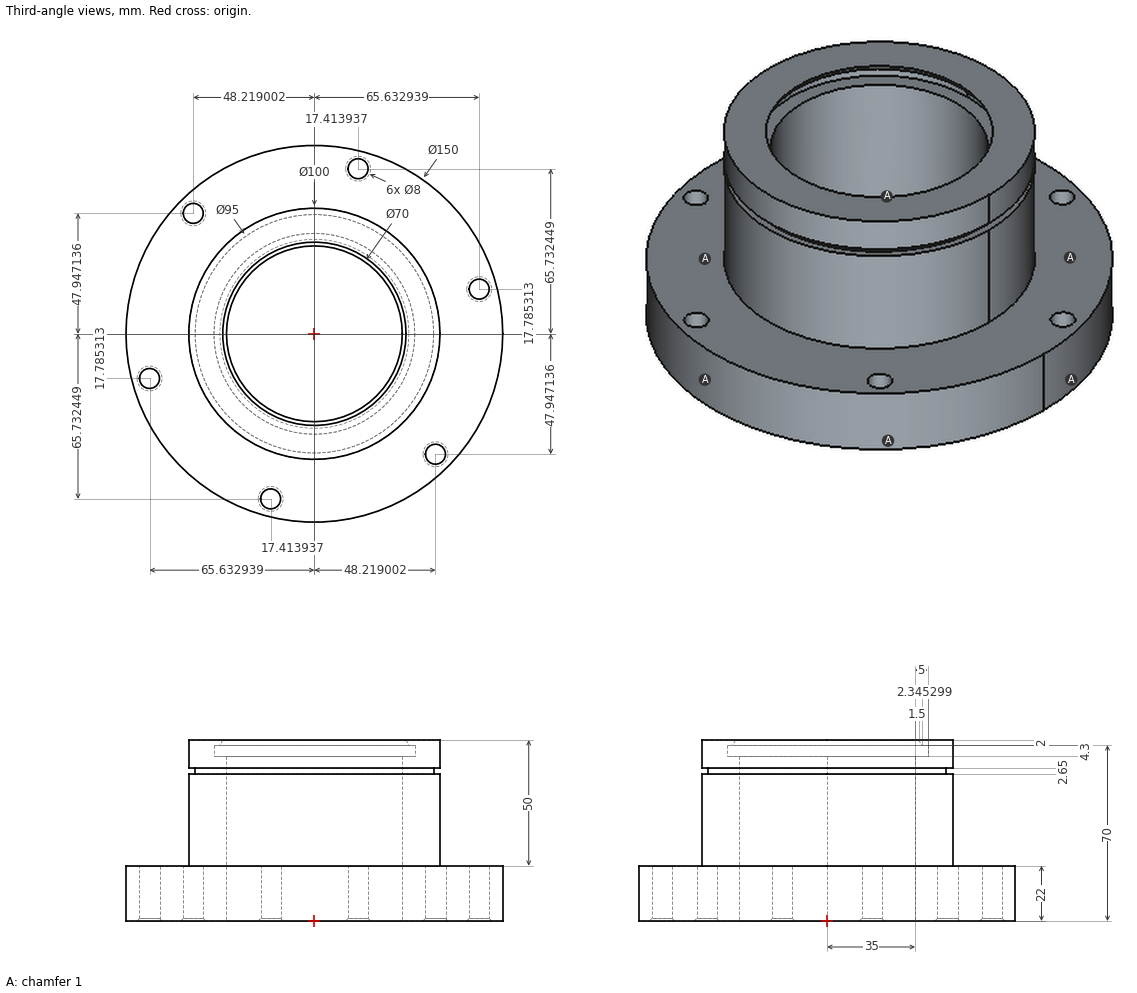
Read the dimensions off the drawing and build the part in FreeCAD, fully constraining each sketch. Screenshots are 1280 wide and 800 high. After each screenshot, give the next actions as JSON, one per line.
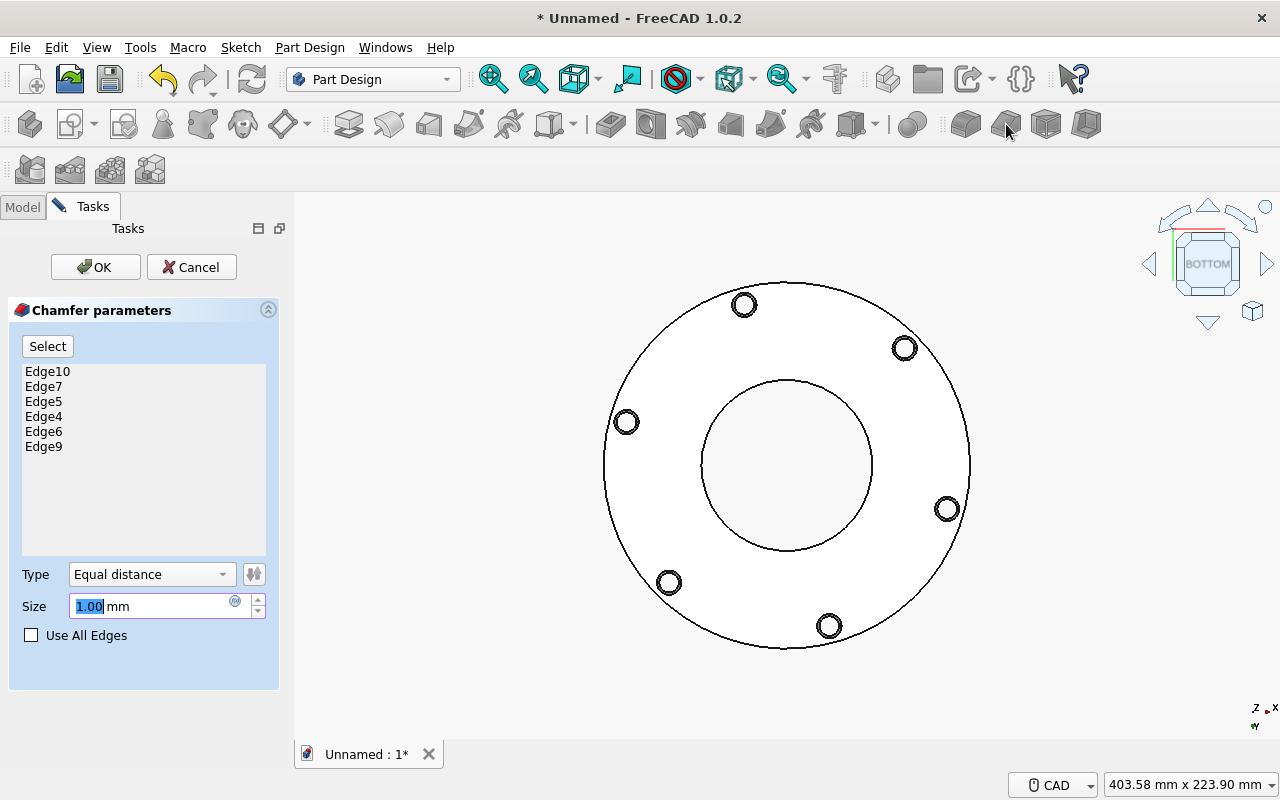
{"action": "type", "text": "1"}
{"action": "key", "text": "Tab"}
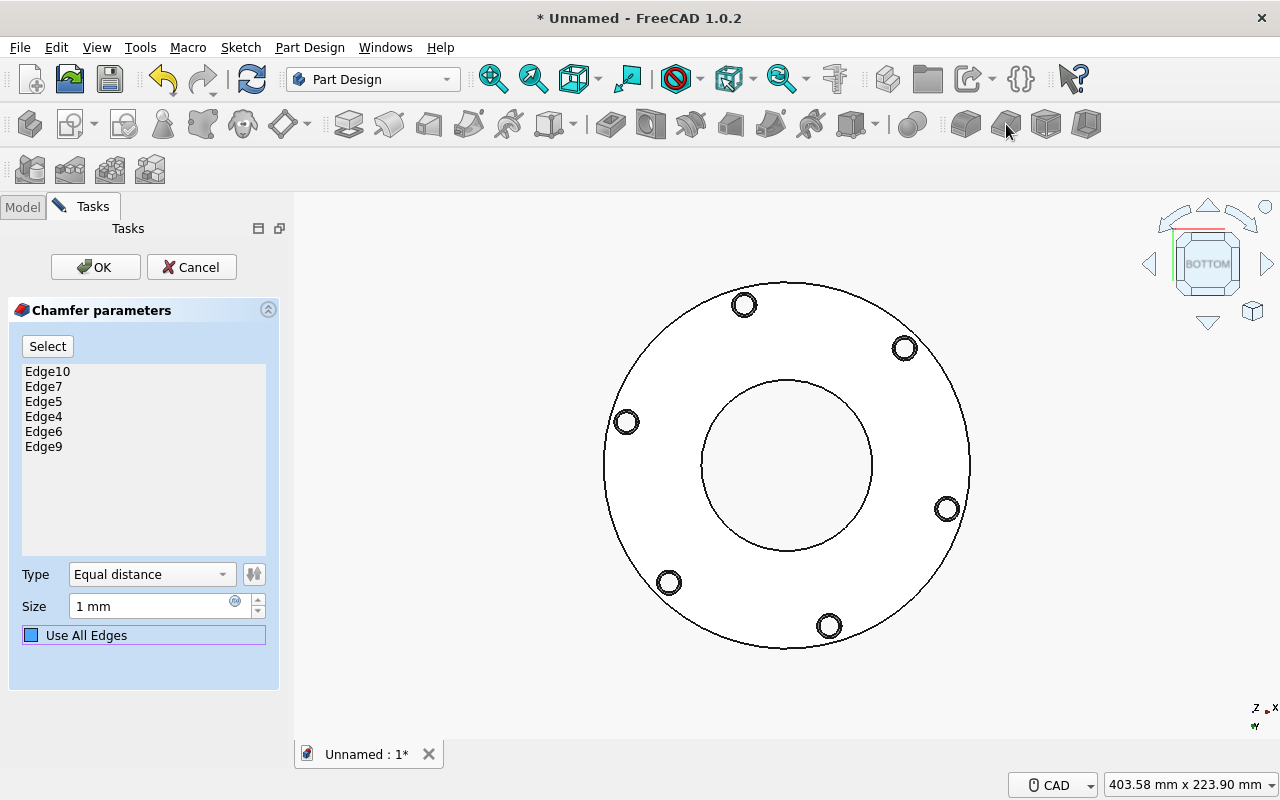
{"action": "left_click", "coordinate": [96, 267]}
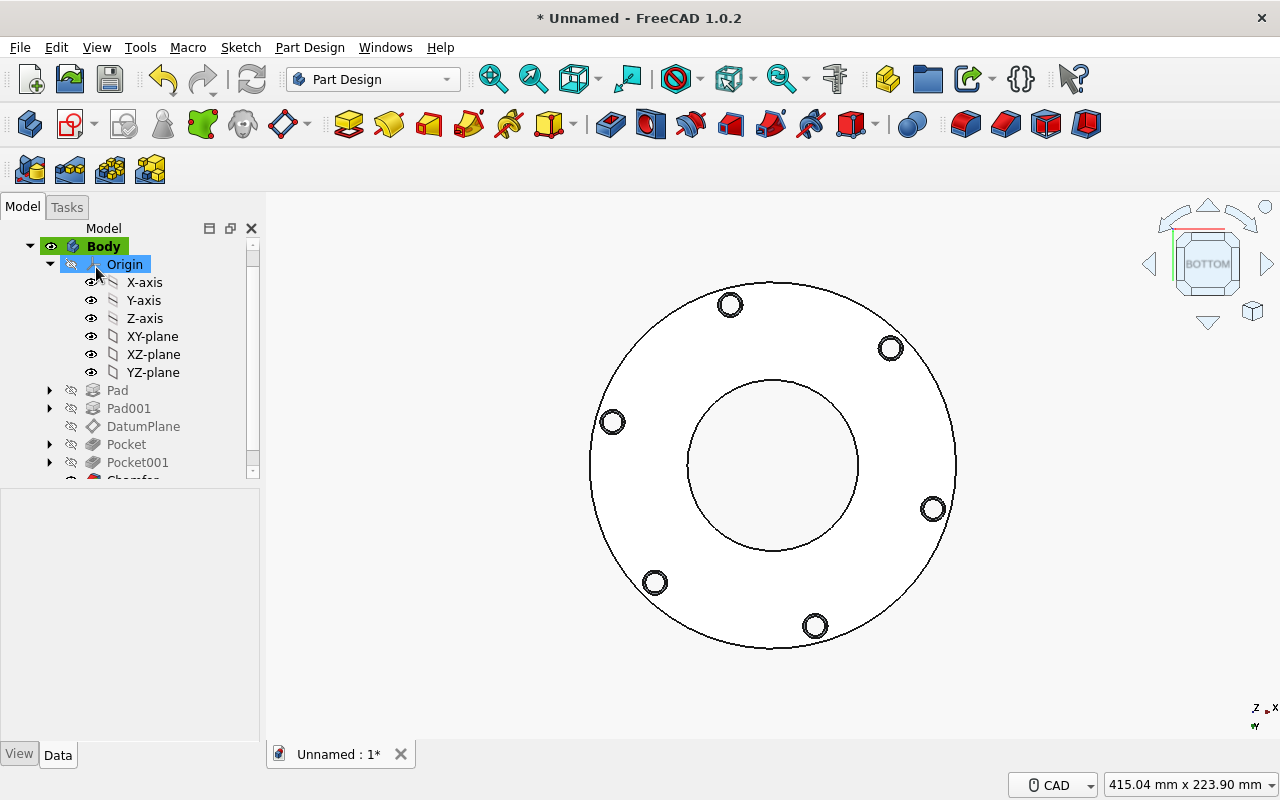
{"action": "left_click", "coordinate": [70, 124]}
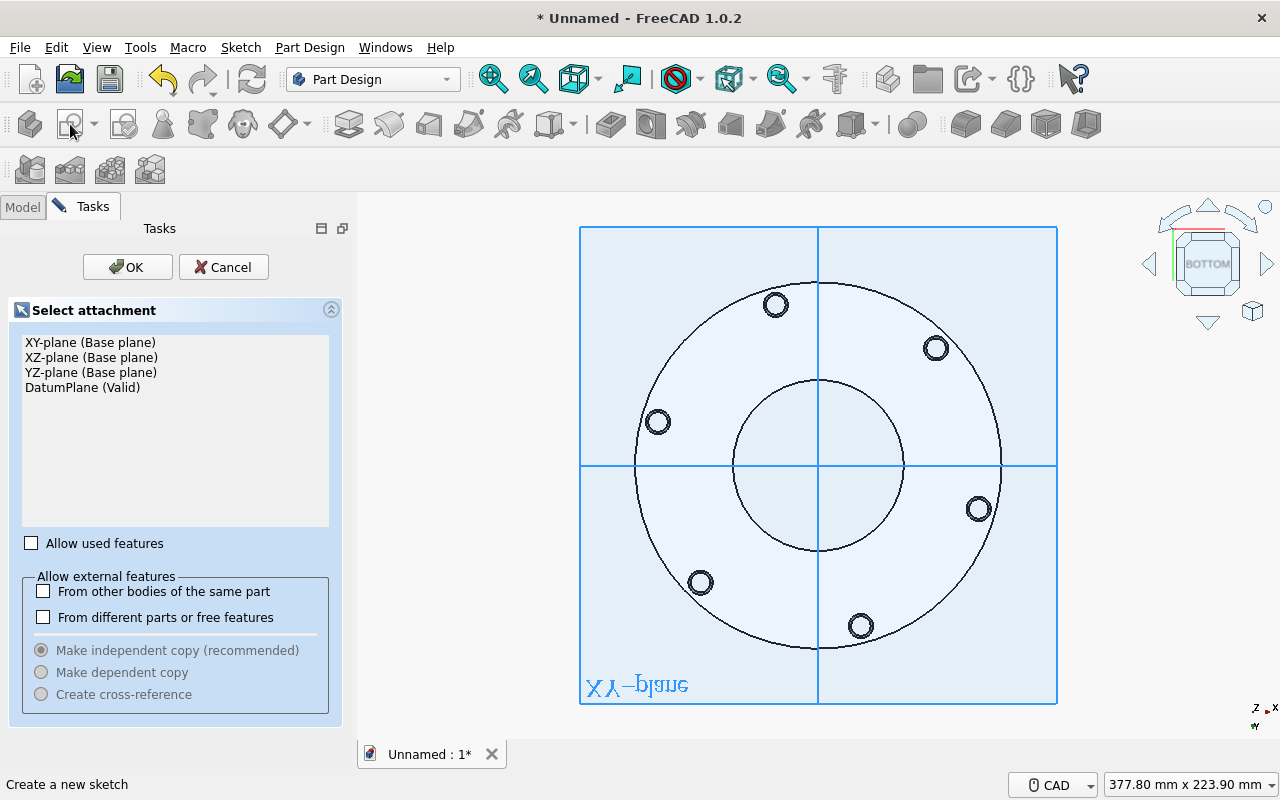
{"action": "left_click", "coordinate": [82, 372]}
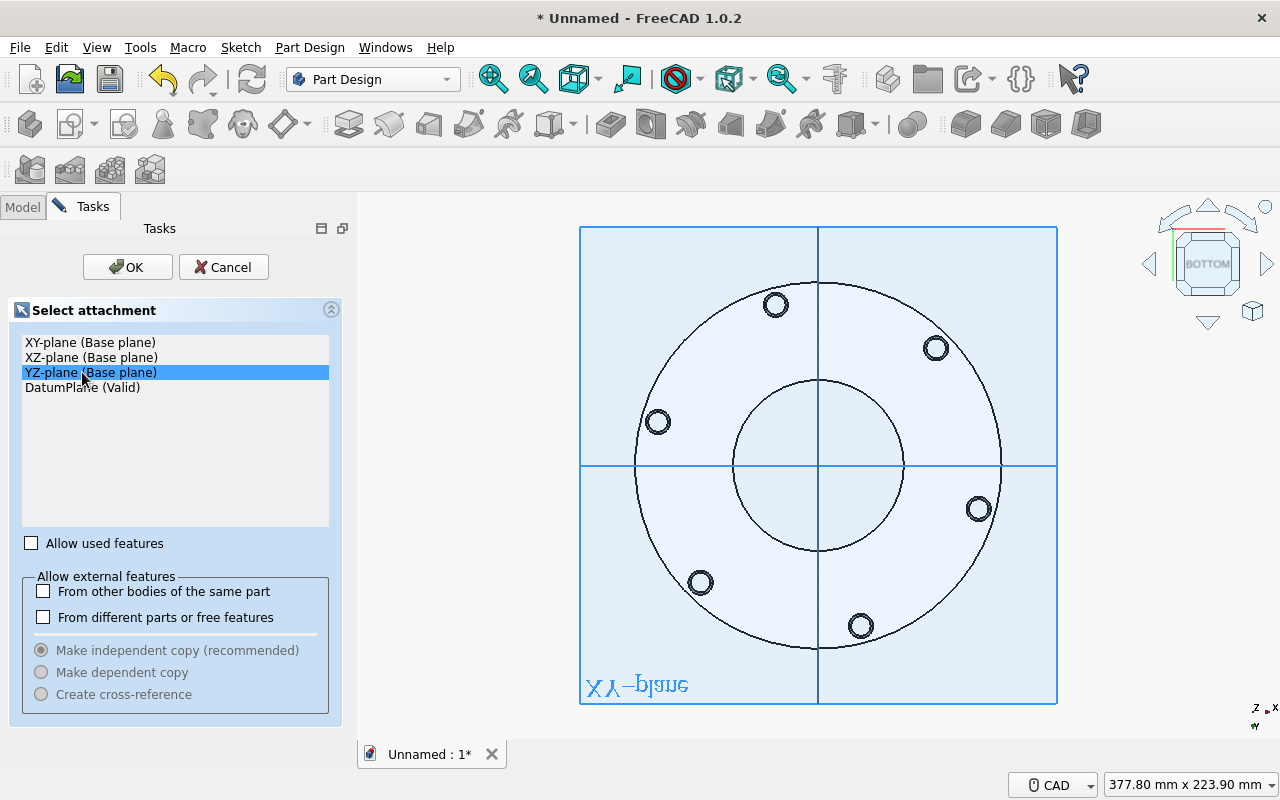
{"action": "left_click", "coordinate": [128, 267]}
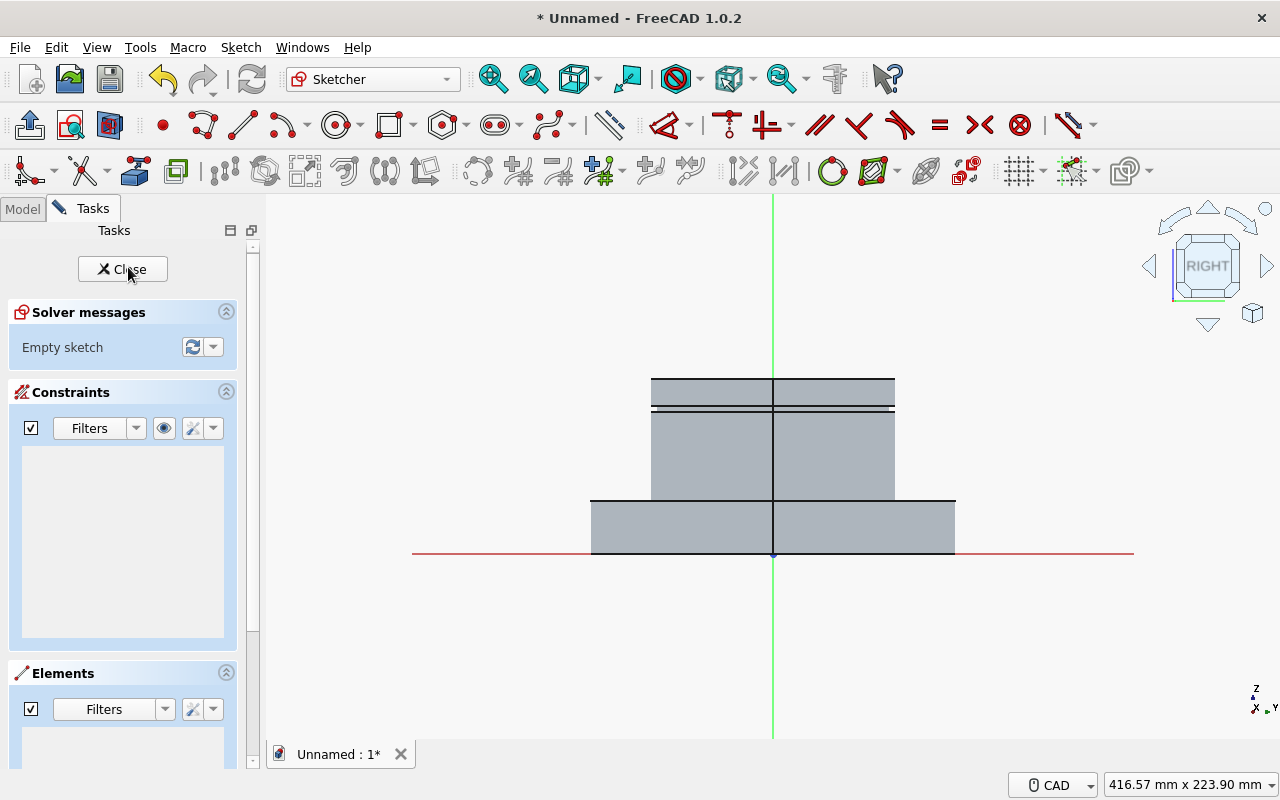
{"action": "left_click", "coordinate": [110, 126]}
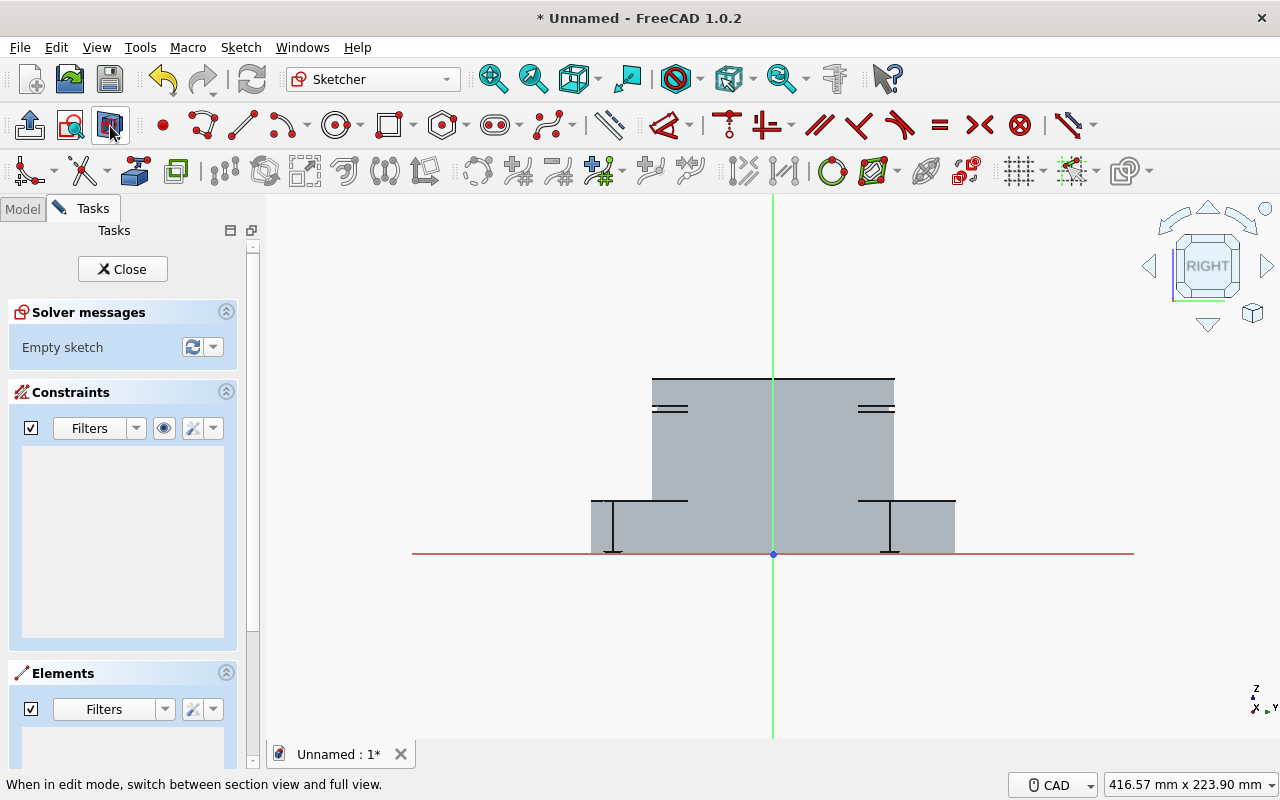
{"action": "scroll", "coordinate": [873, 382], "scroll_direction": "up", "scroll_amount": 15}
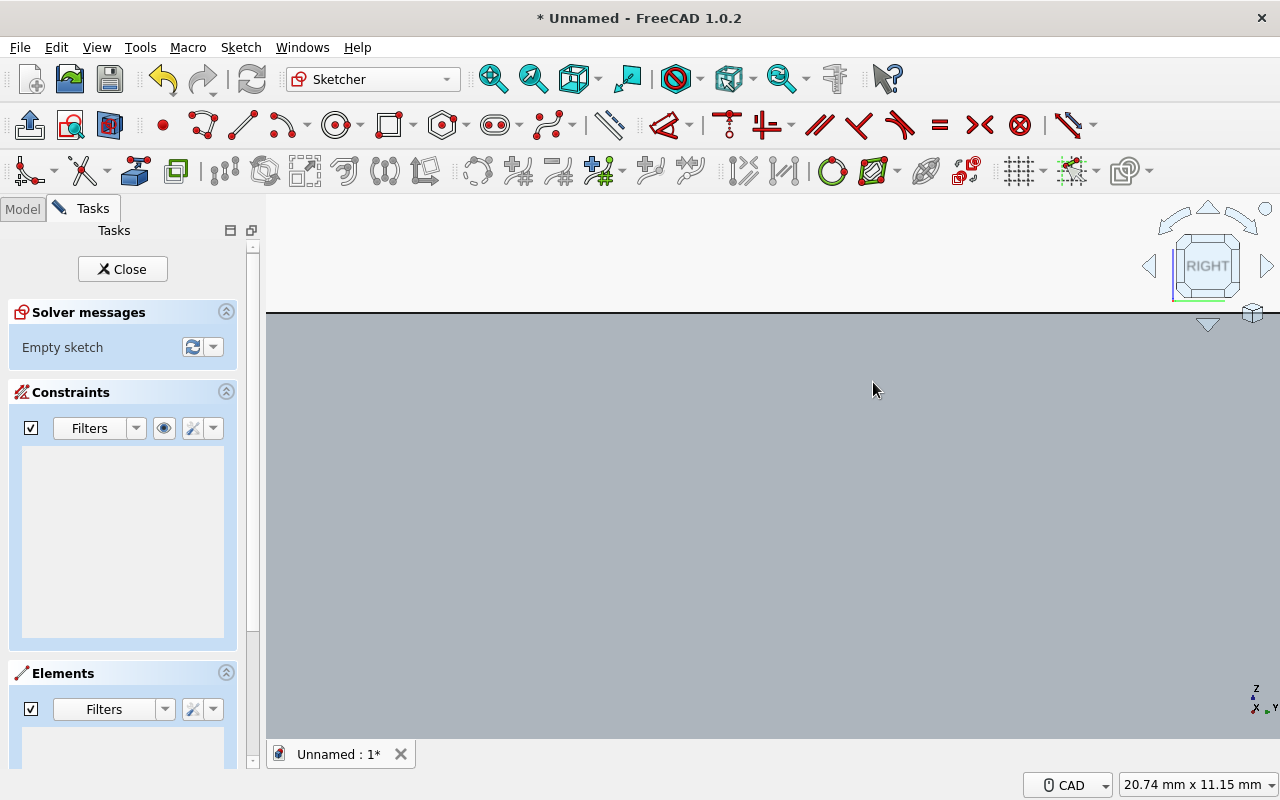
{"action": "left_click", "coordinate": [204, 126]}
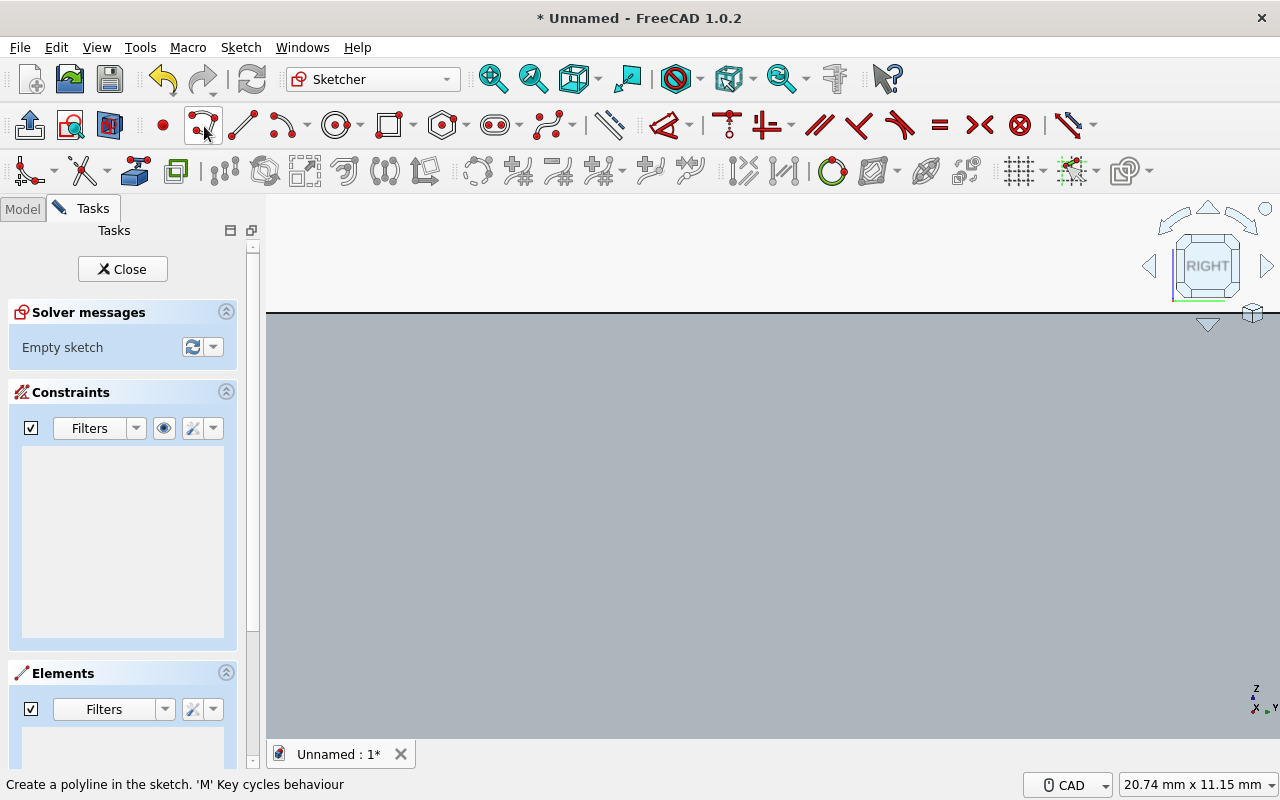
{"action": "left_click", "coordinate": [564, 621]}
{"action": "left_click", "coordinate": [809, 621]}
{"action": "left_click", "coordinate": [809, 410]}
{"action": "left_click", "coordinate": [694, 410]}
{"action": "left_click", "coordinate": [638, 313]}
{"action": "left_click", "coordinate": [564, 313]}
{"action": "left_click", "coordinate": [564, 622]}
{"action": "key", "text": "Escape"}
{"action": "key", "text": "Escape"}